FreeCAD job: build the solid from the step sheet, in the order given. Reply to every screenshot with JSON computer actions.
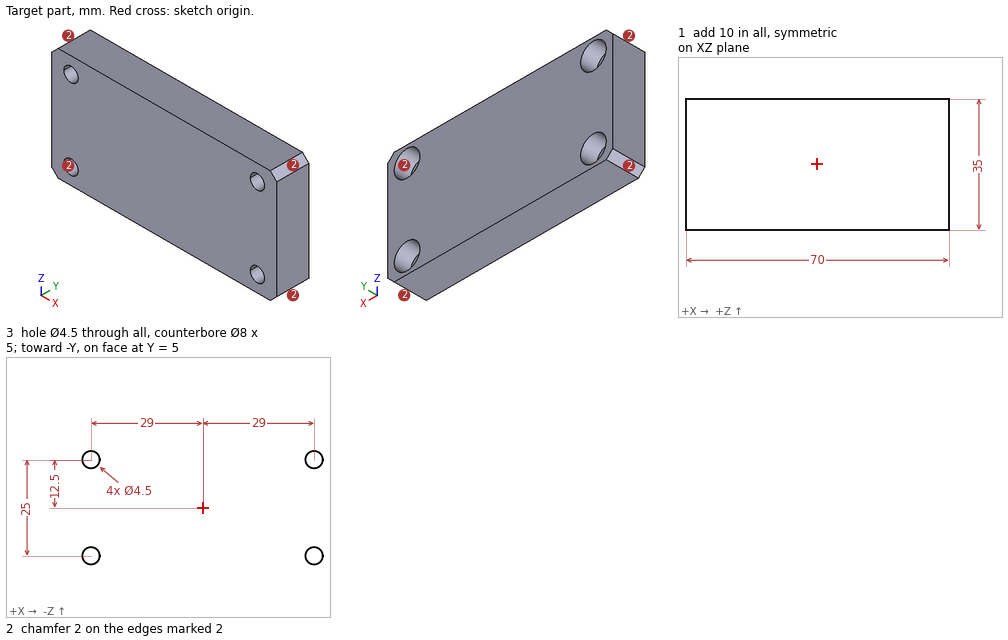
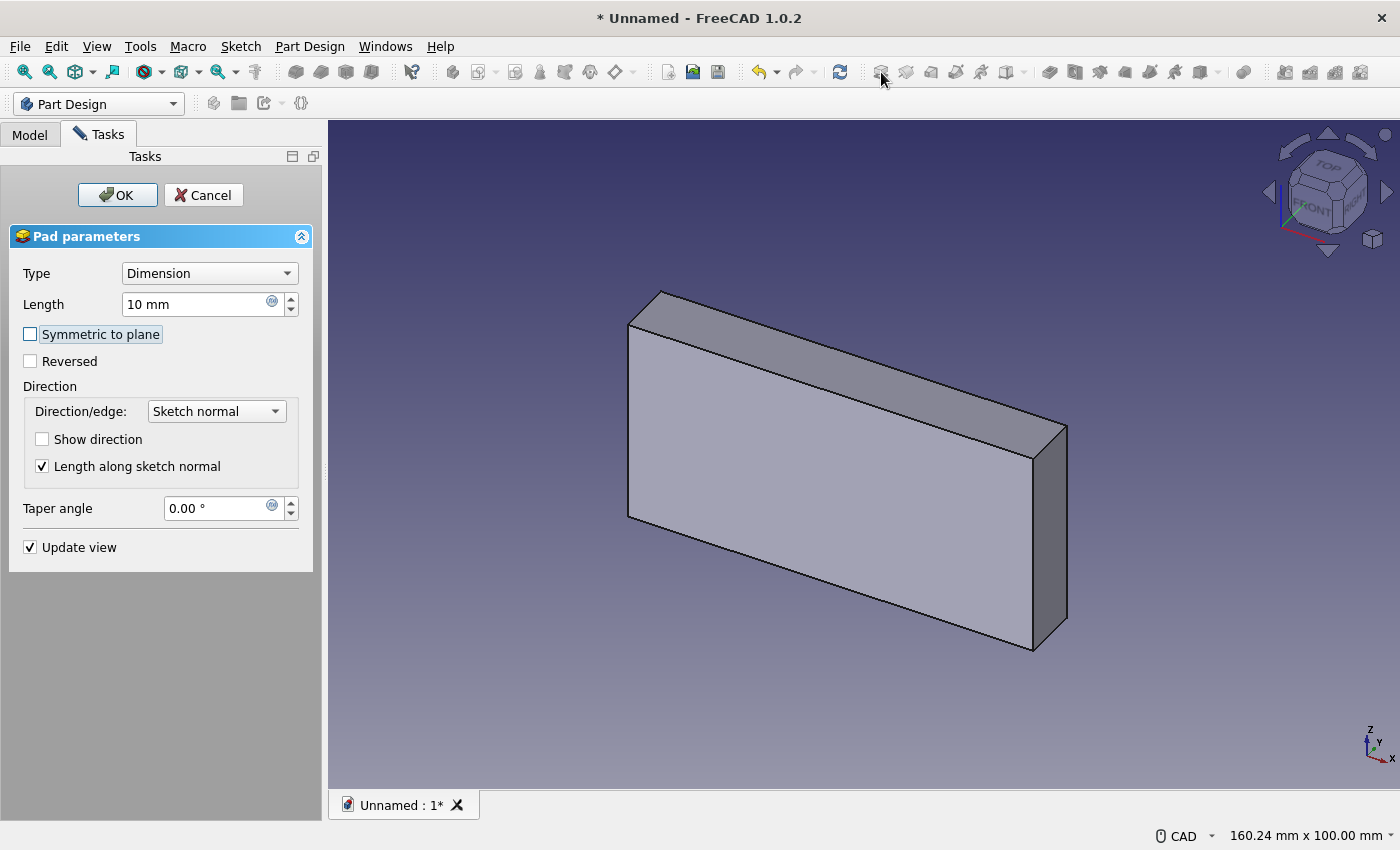
{"action": "left_click", "coordinate": [31, 334]}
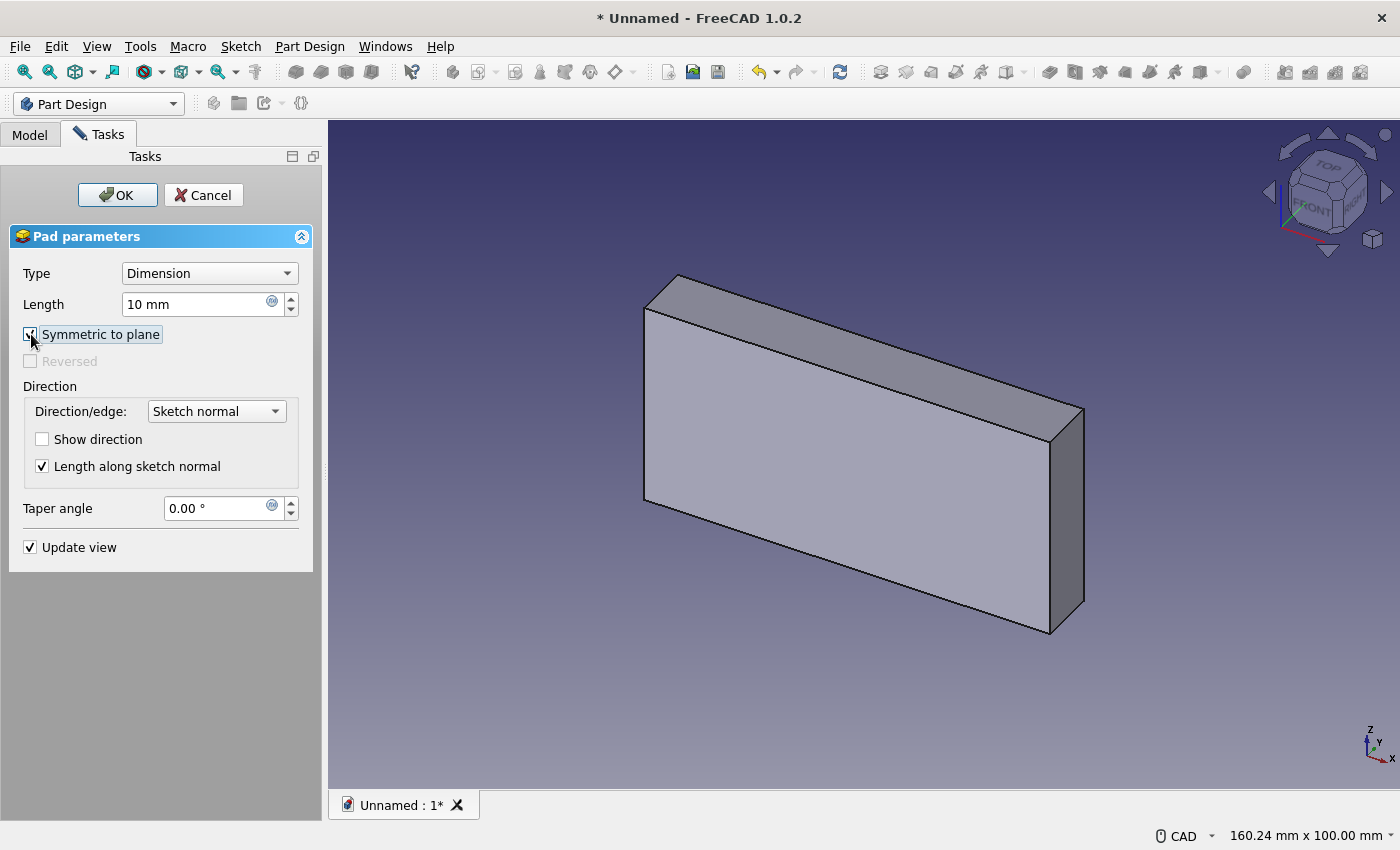
{"action": "left_click", "coordinate": [118, 195]}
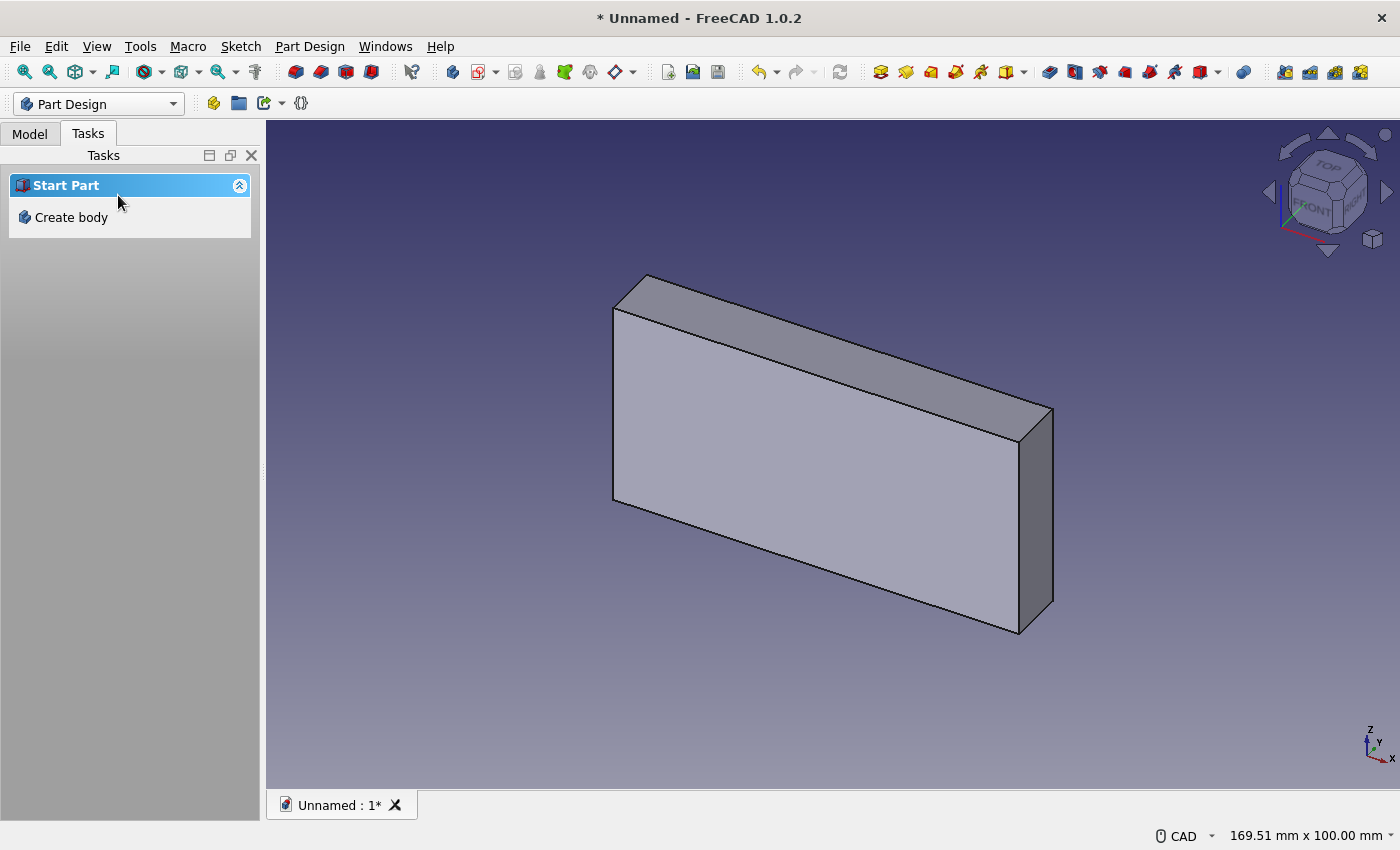
{"action": "left_click", "coordinate": [1036, 425]}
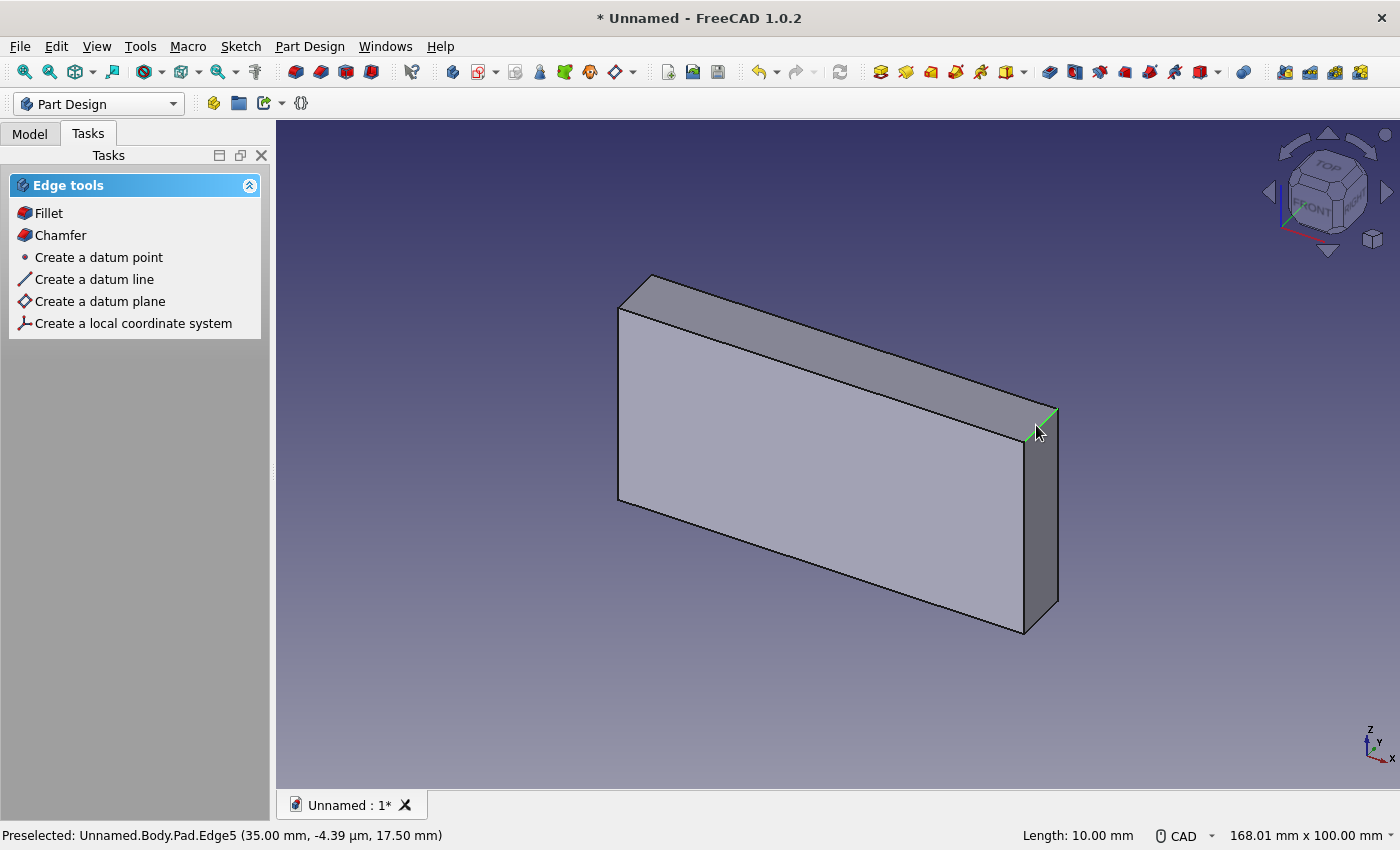
{"action": "key", "text": "0"}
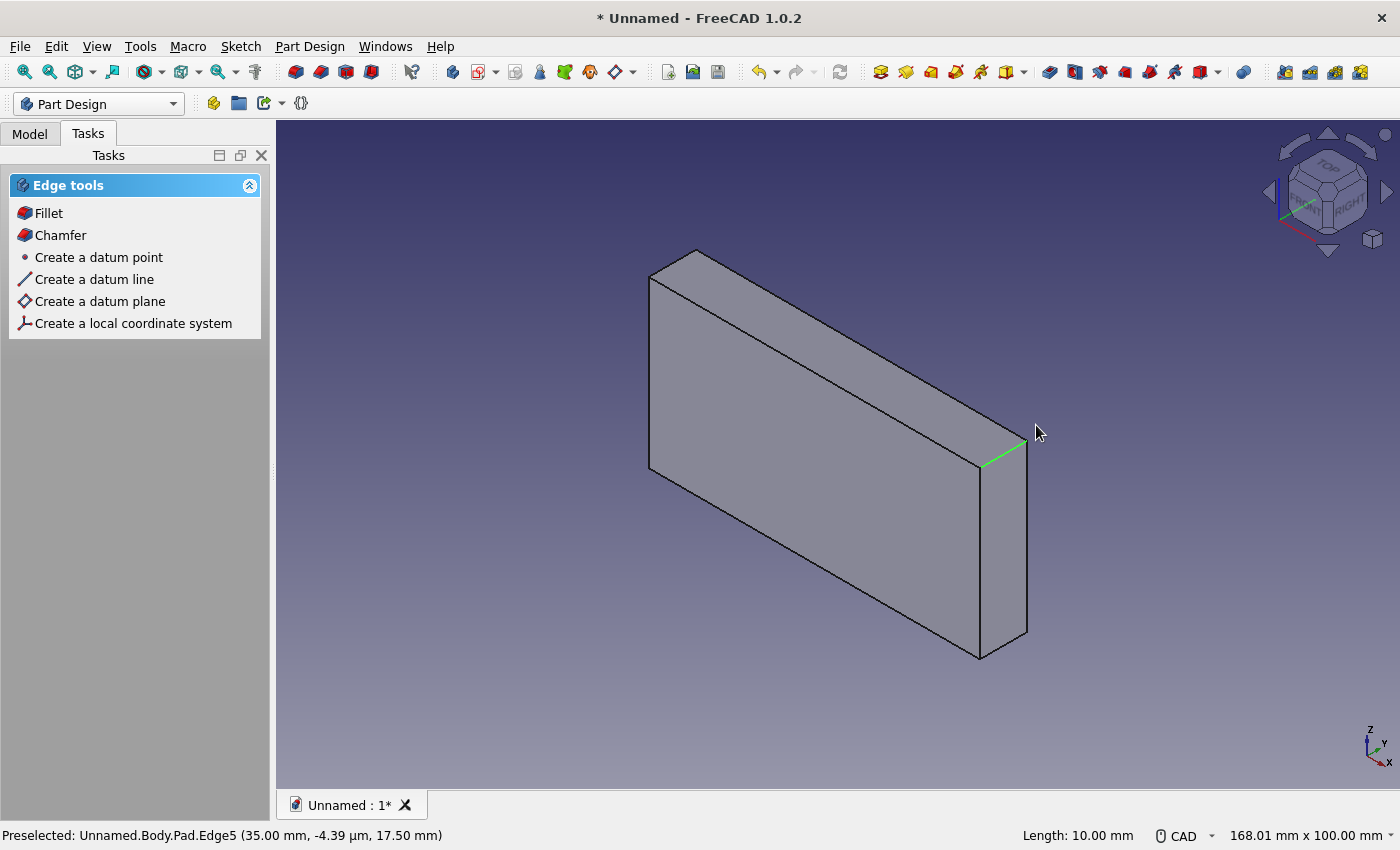
{"action": "key", "text": "2"}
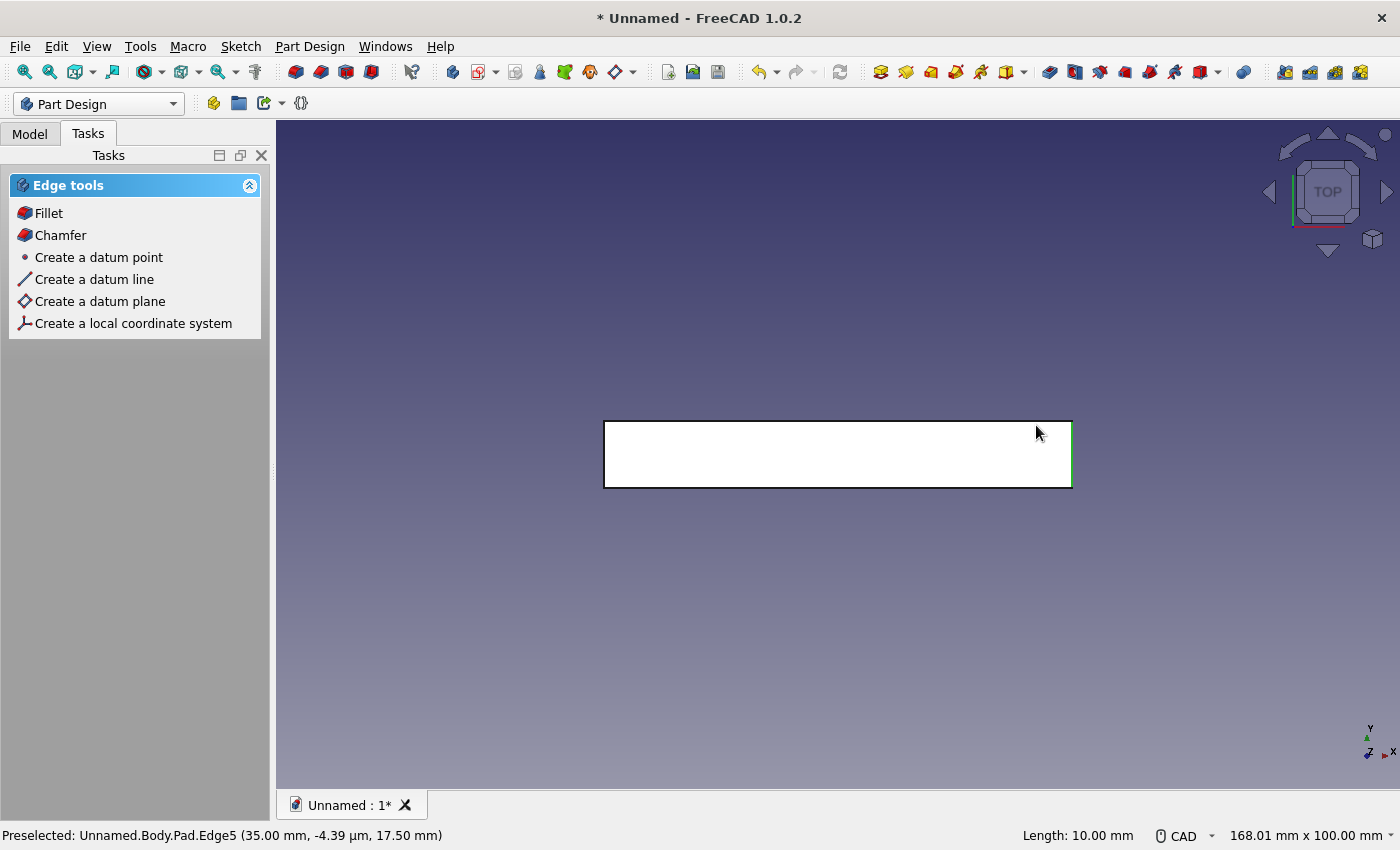
{"action": "left_click", "coordinate": [25, 72]}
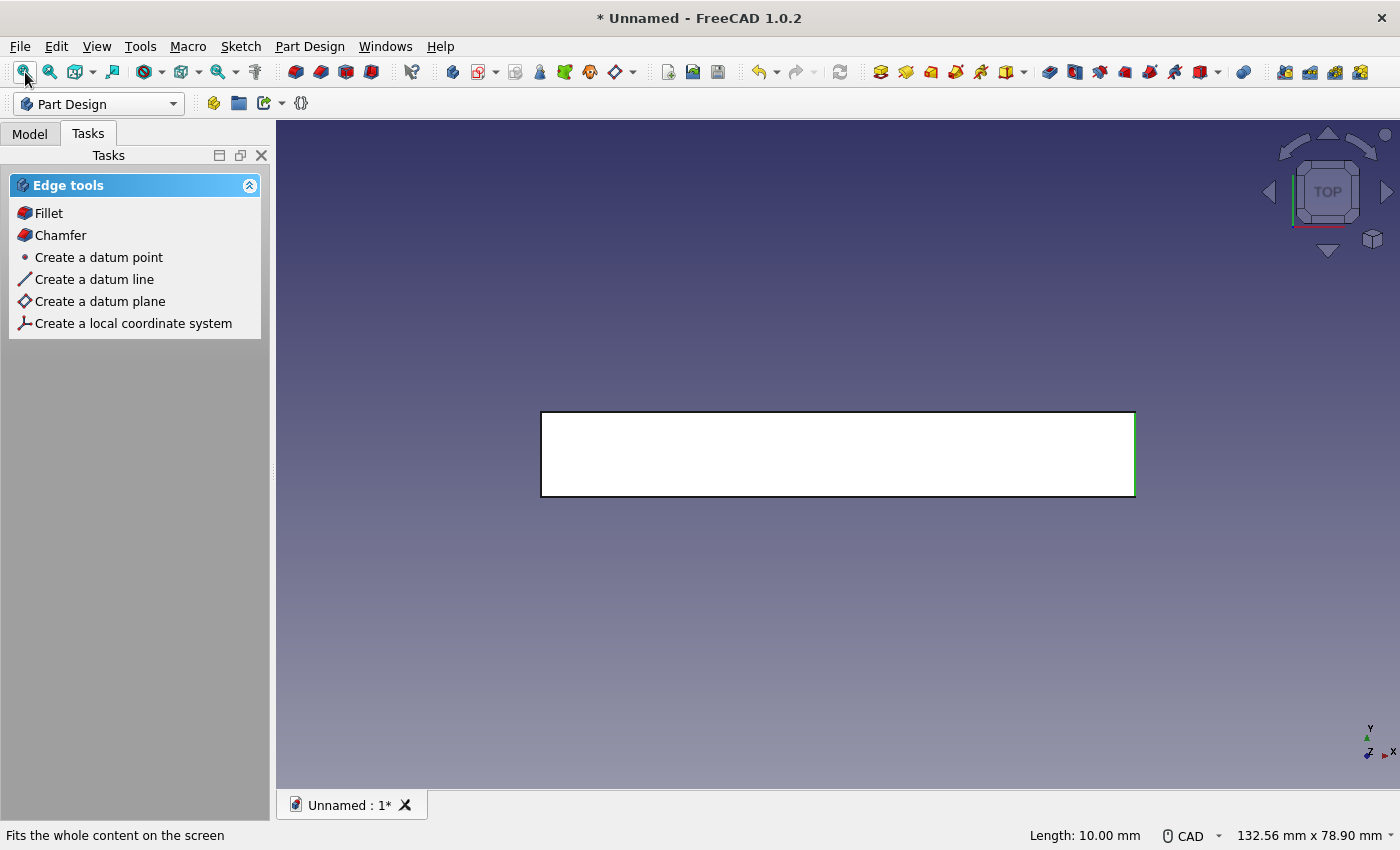
{"action": "left_click", "coordinate": [541, 453], "text": "ctrl"}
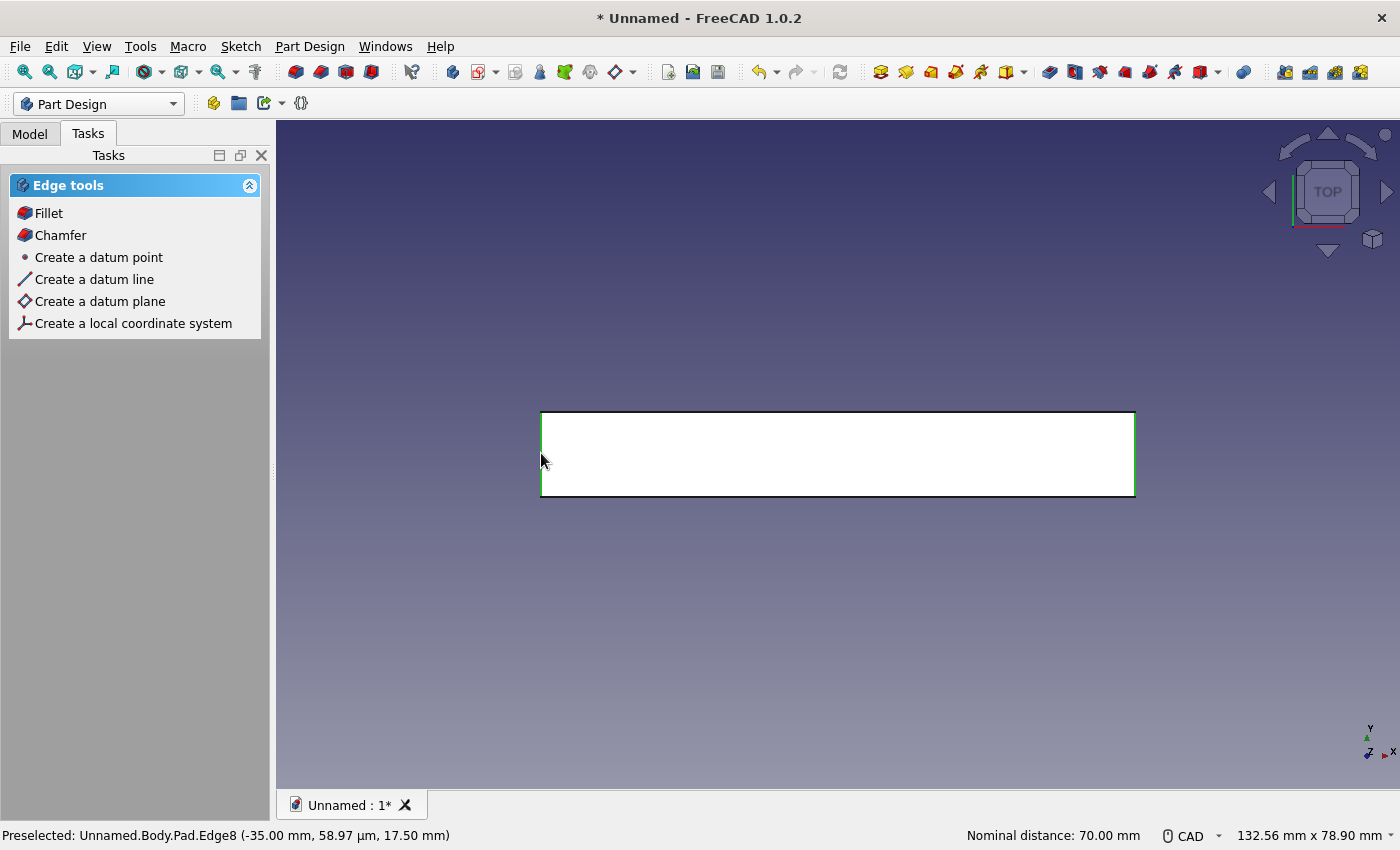
{"action": "key", "text": "1"}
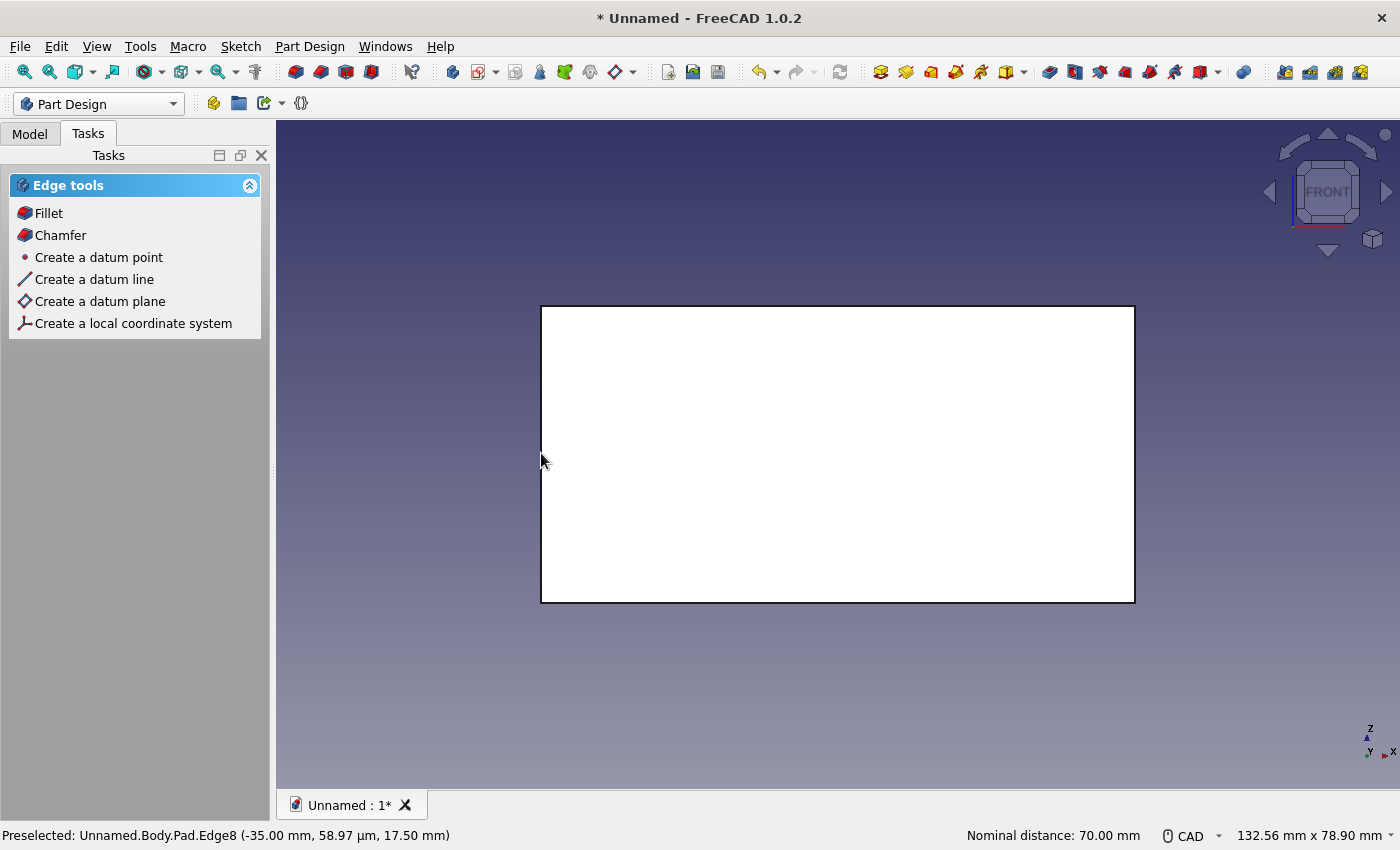
{"action": "key", "text": "3"}